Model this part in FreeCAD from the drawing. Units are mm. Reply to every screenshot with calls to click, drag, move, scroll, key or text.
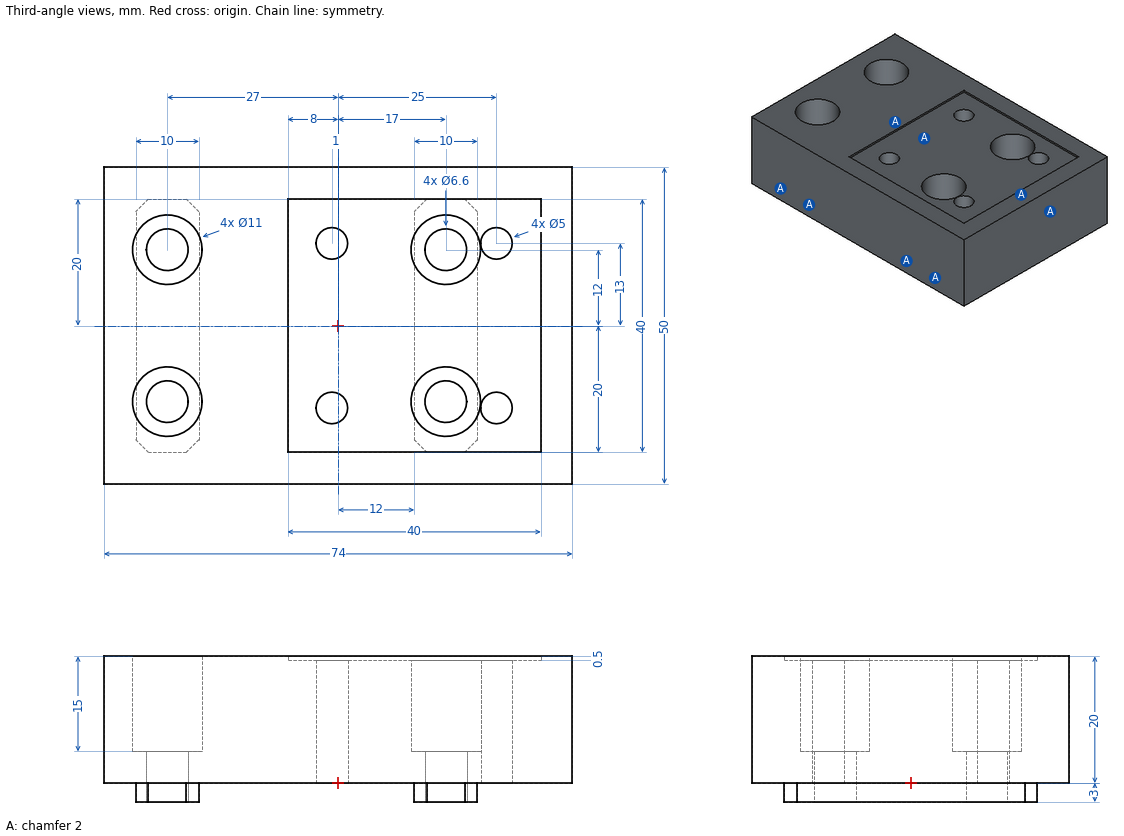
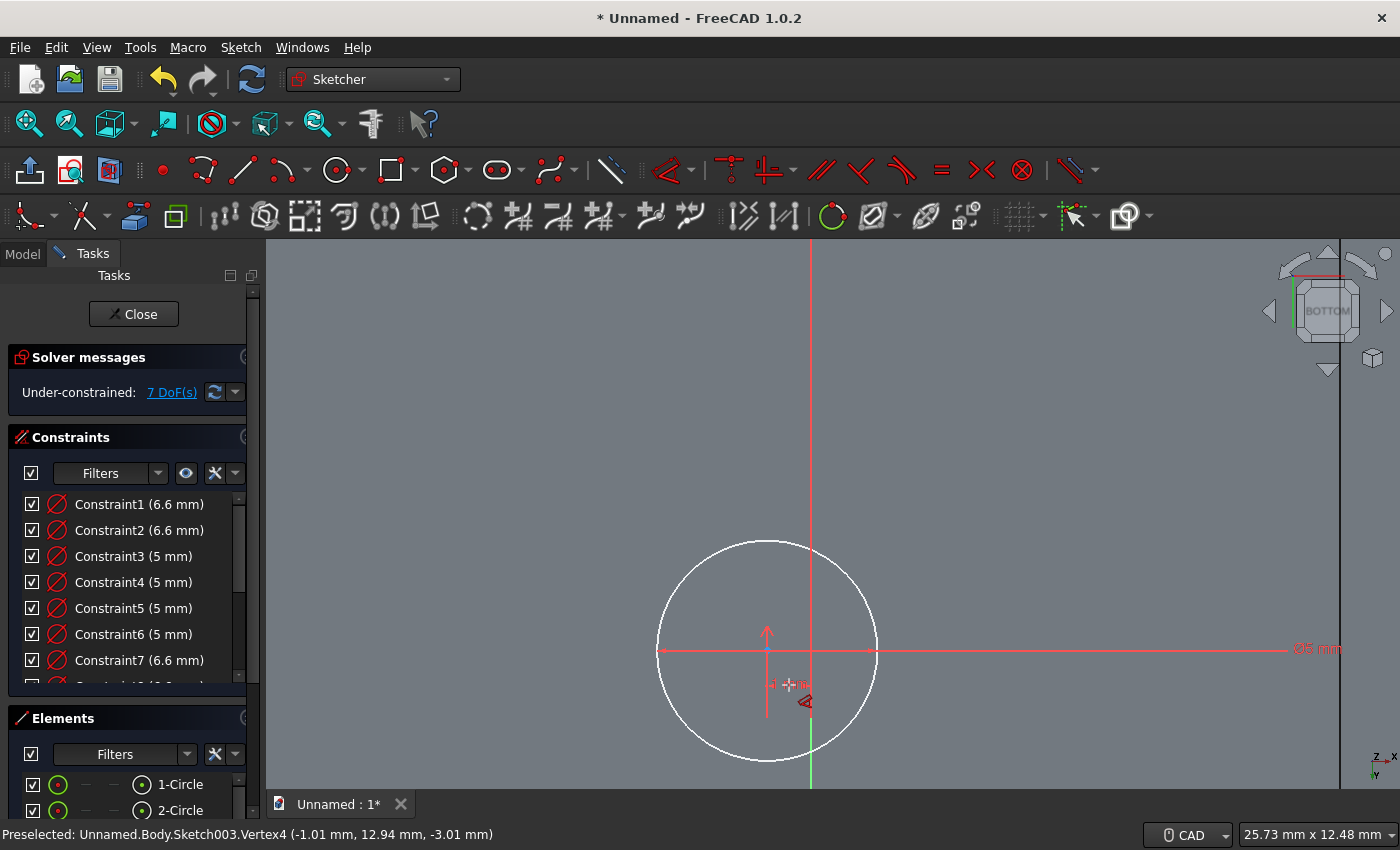
scroll(769, 656, down, 7)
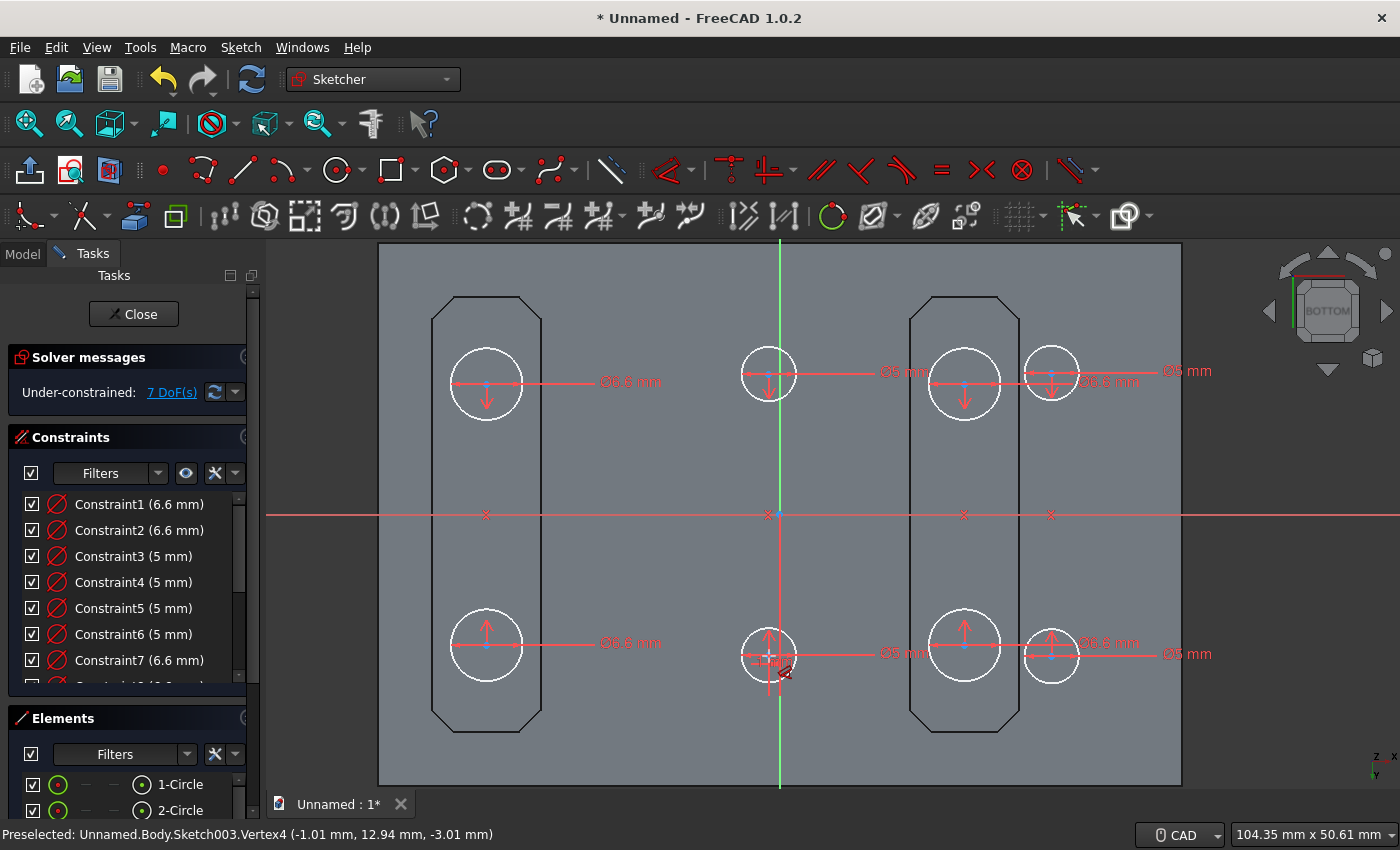
click(965, 645)
click(872, 679)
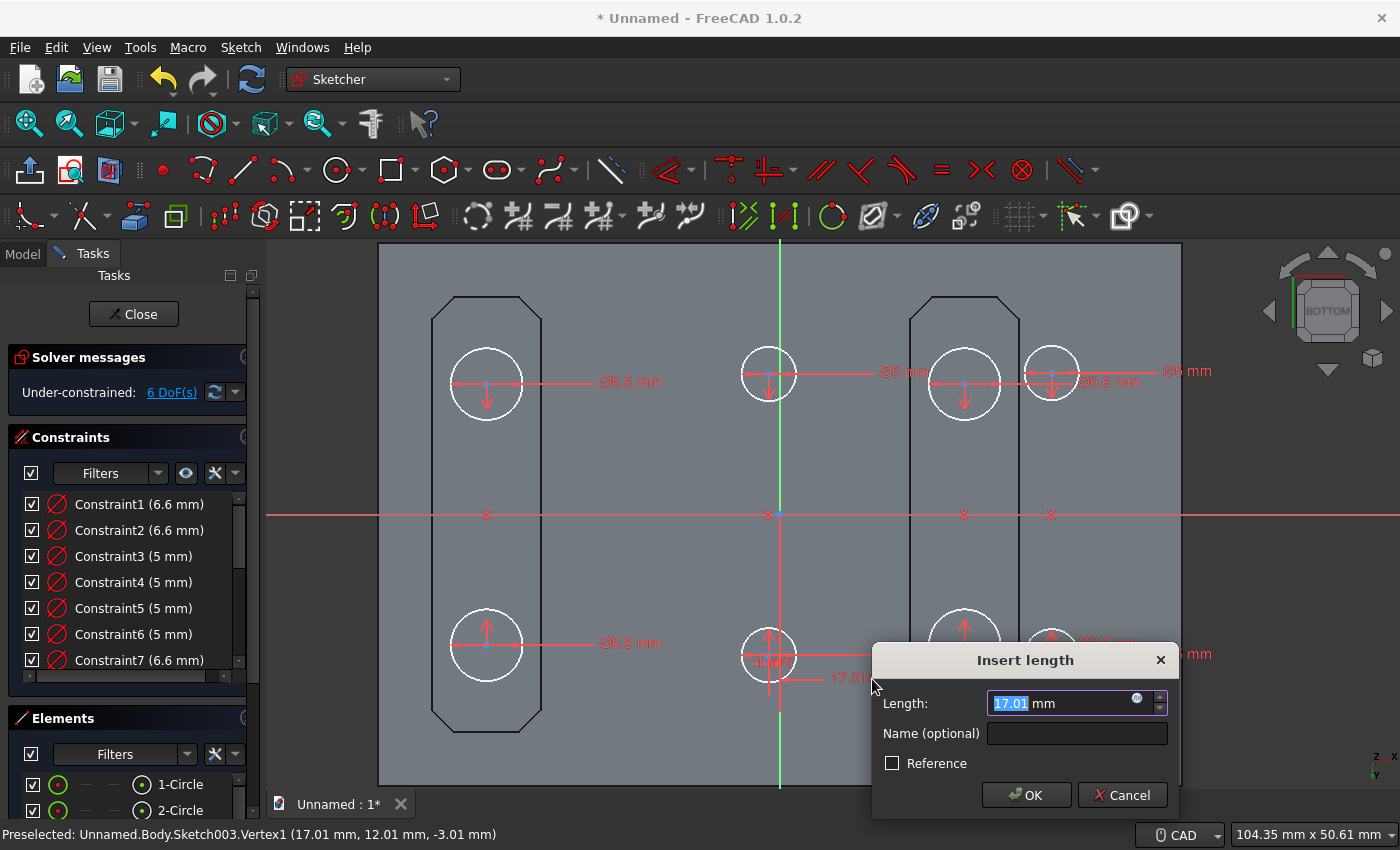
text(17)
key(Return)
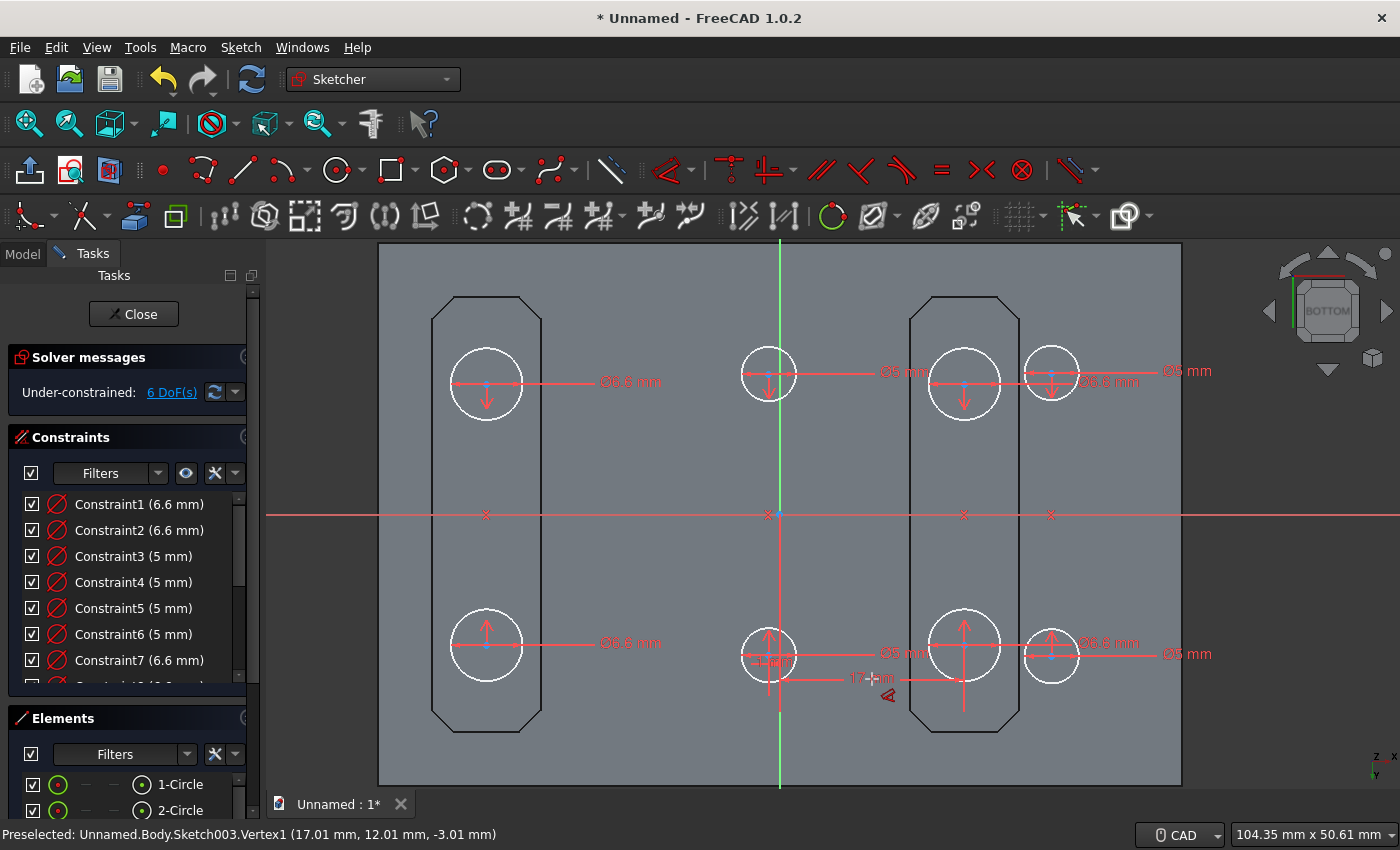
click(964, 645)
click(998, 580)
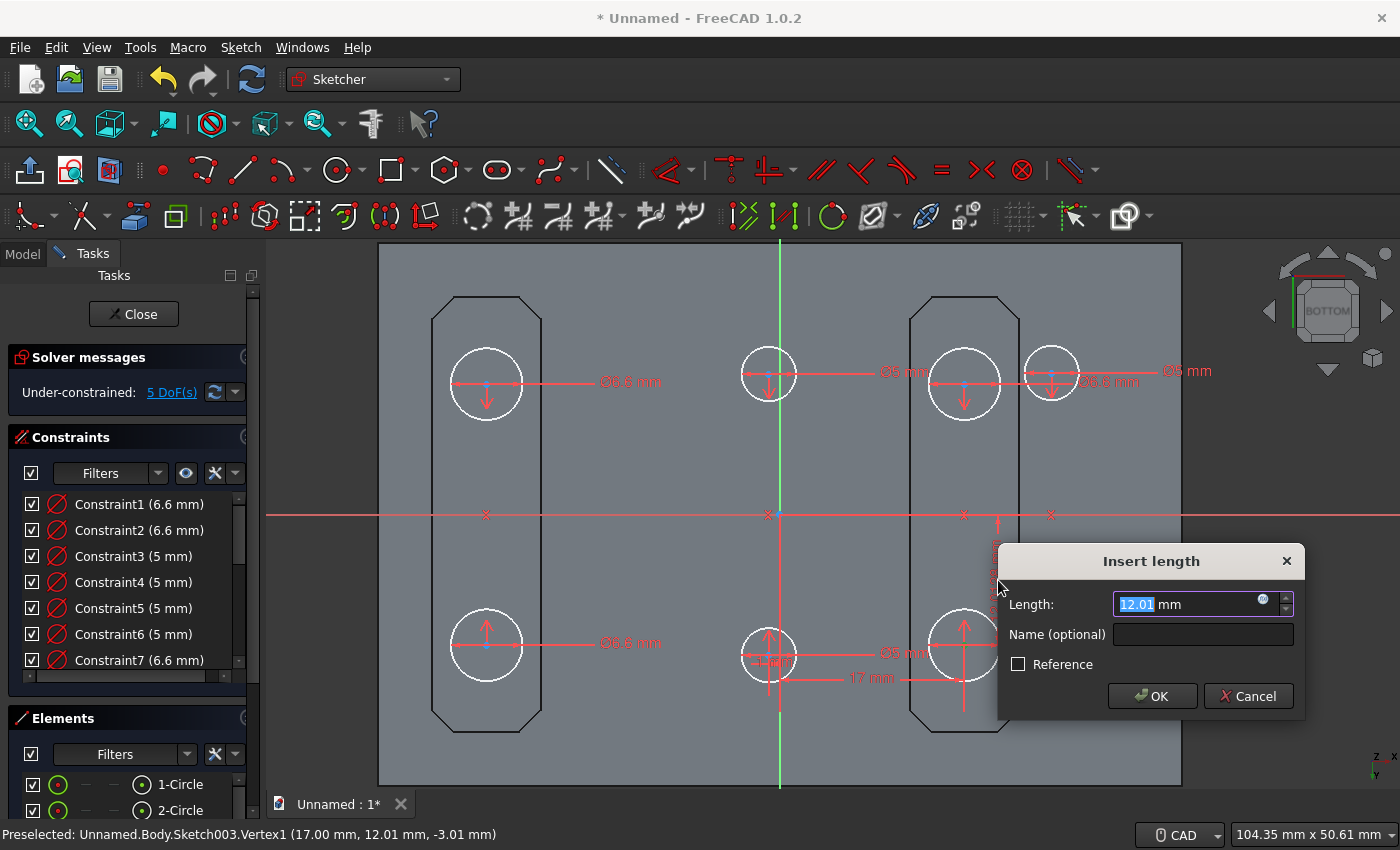
text(12)
key(Return)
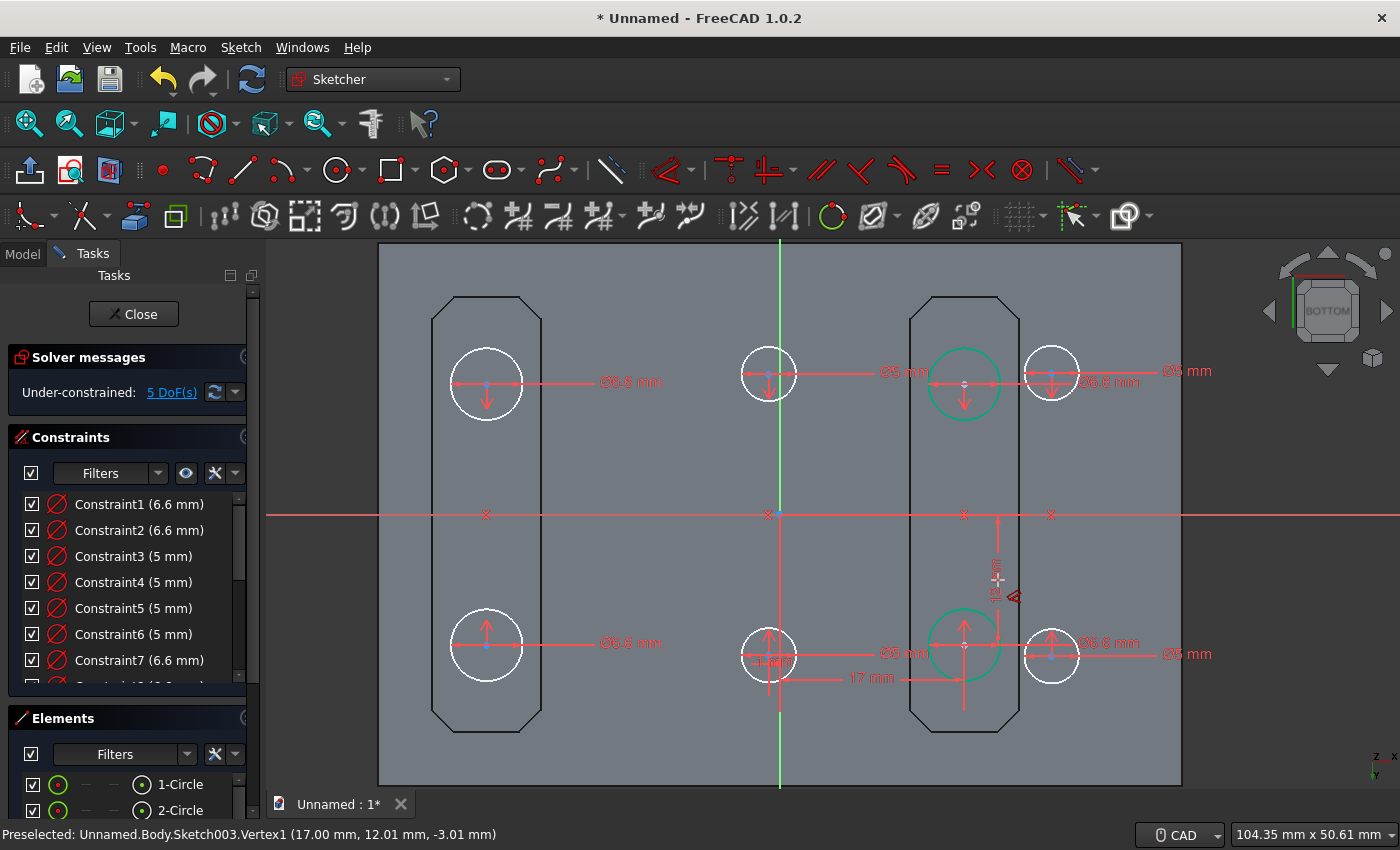
click(487, 645)
click(633, 679)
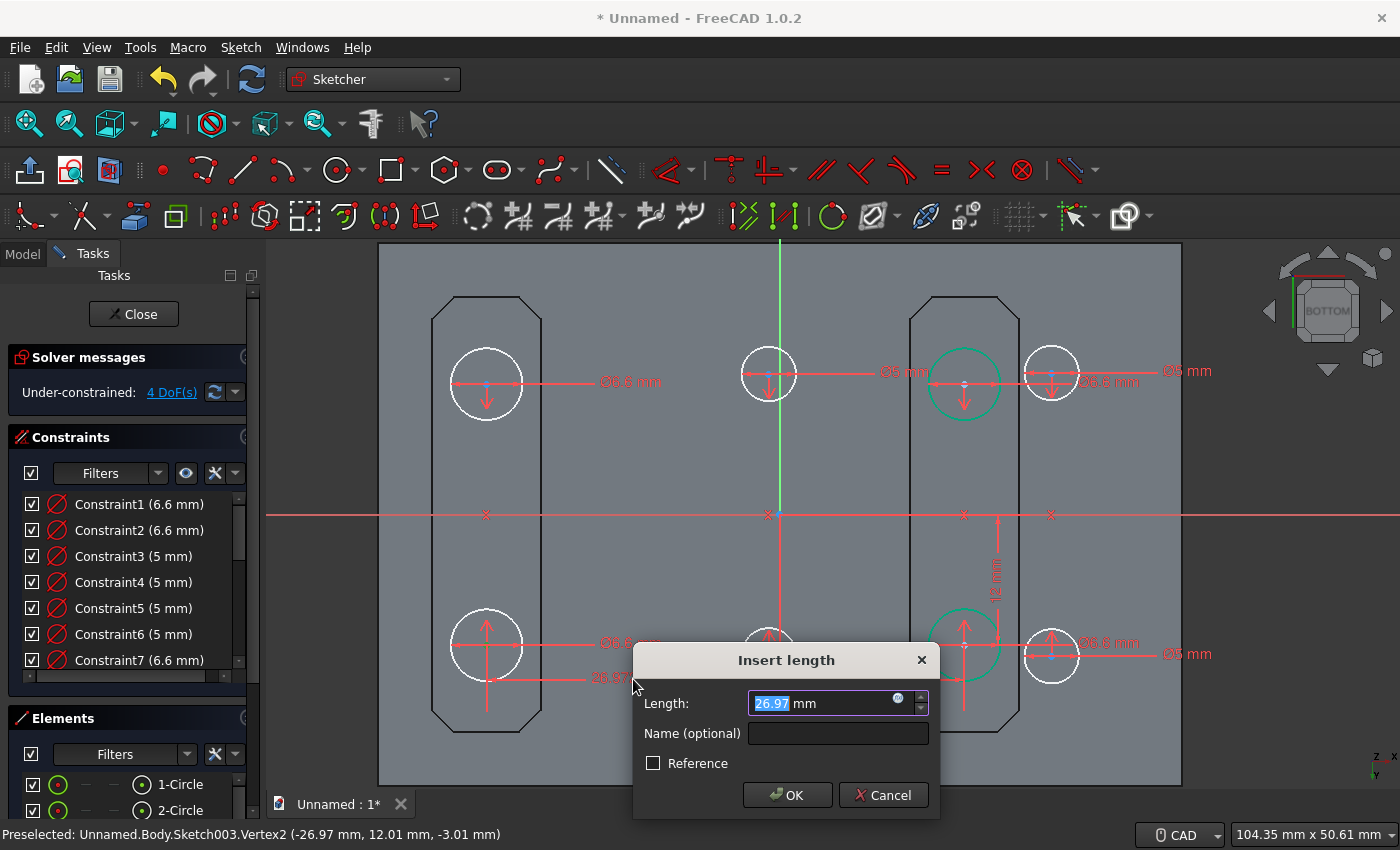
text(27)
key(Return)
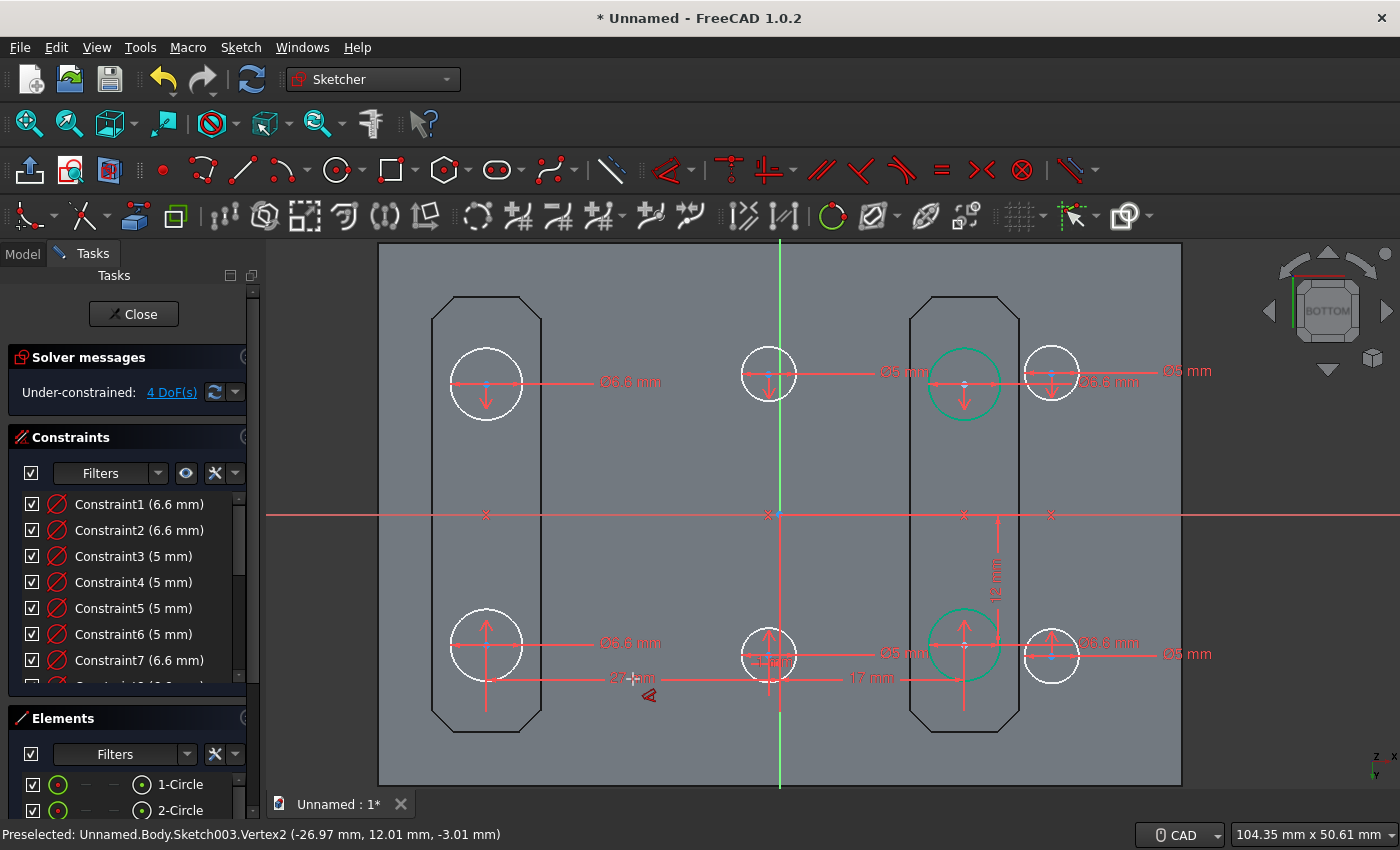
click(486, 645)
click(452, 580)